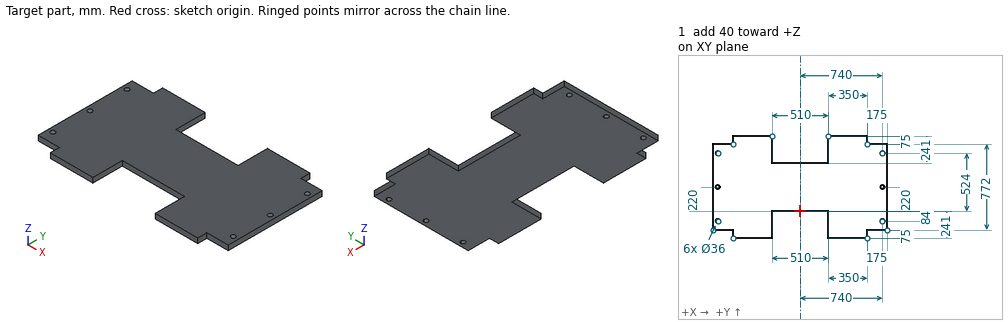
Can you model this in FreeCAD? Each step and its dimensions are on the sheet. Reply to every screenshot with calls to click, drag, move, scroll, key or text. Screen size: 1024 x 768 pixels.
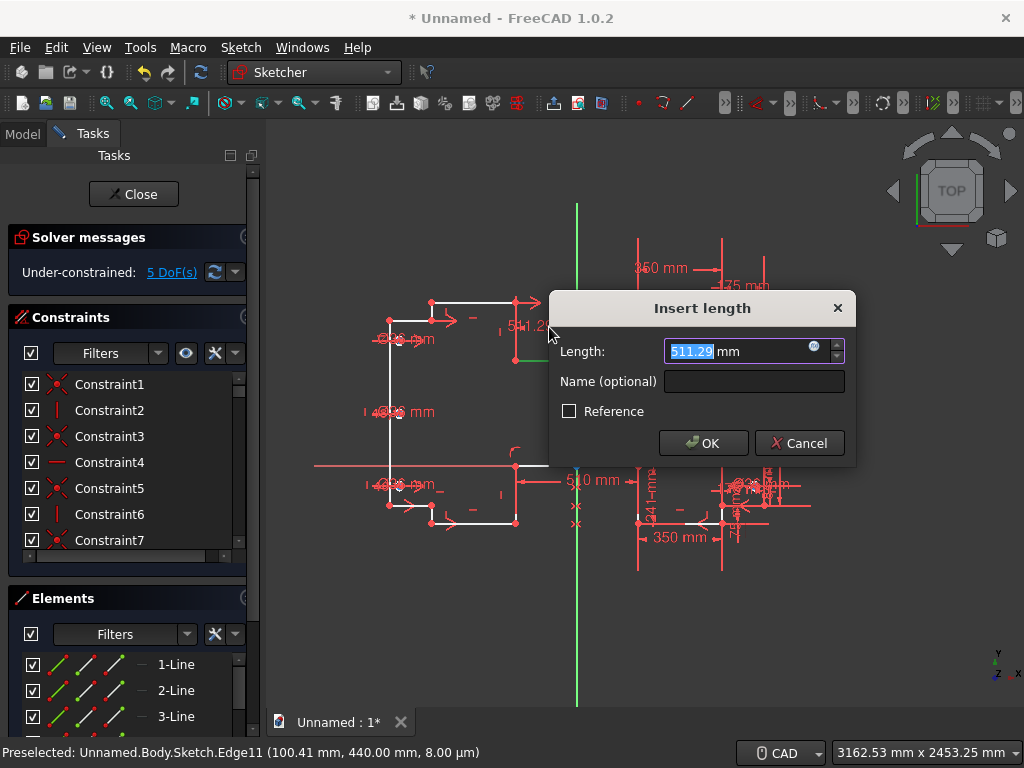
text(510)
key(Return)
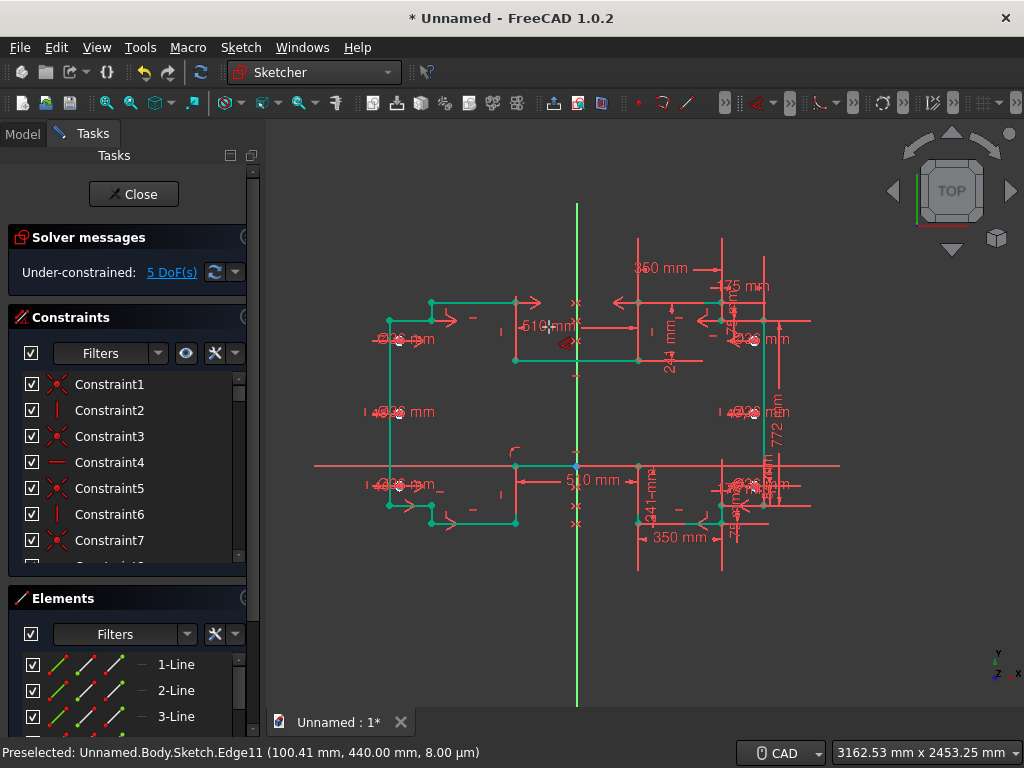
click(754, 486)
click(604, 520)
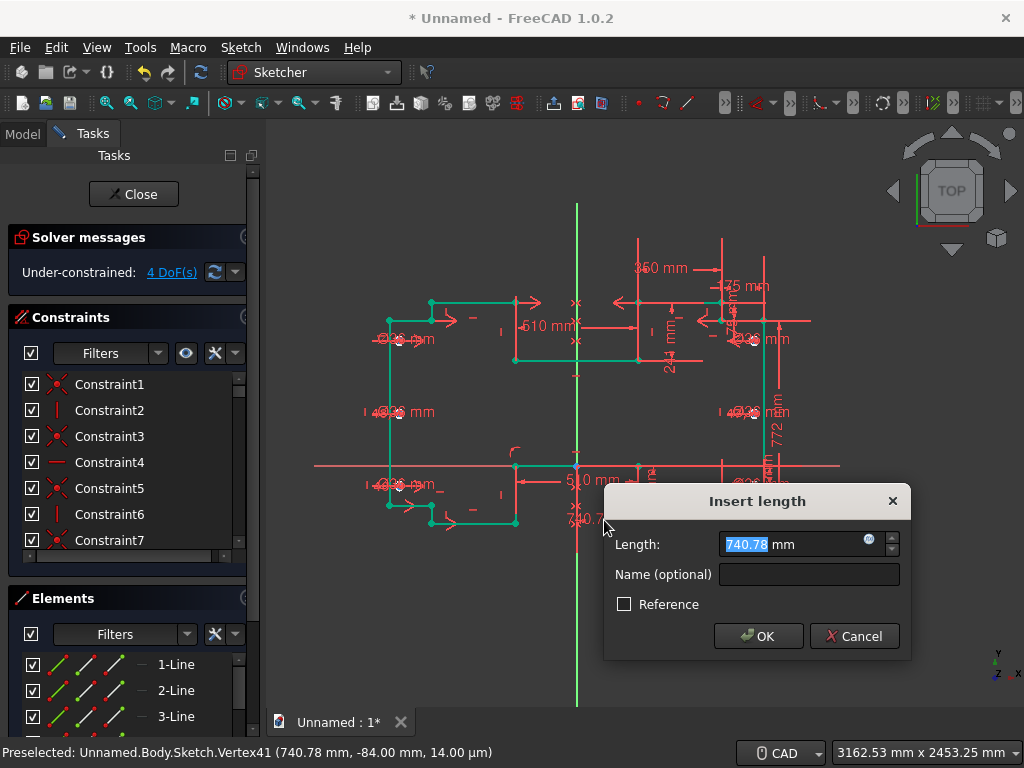
text(740)
key(Return)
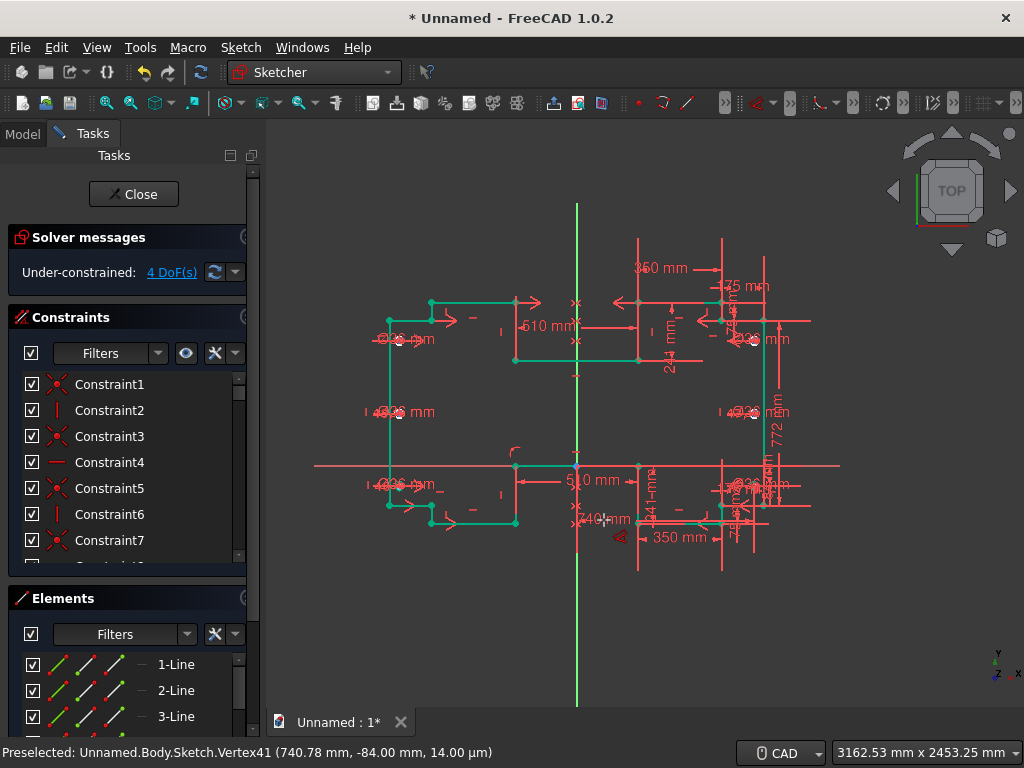
click(754, 414)
click(788, 452)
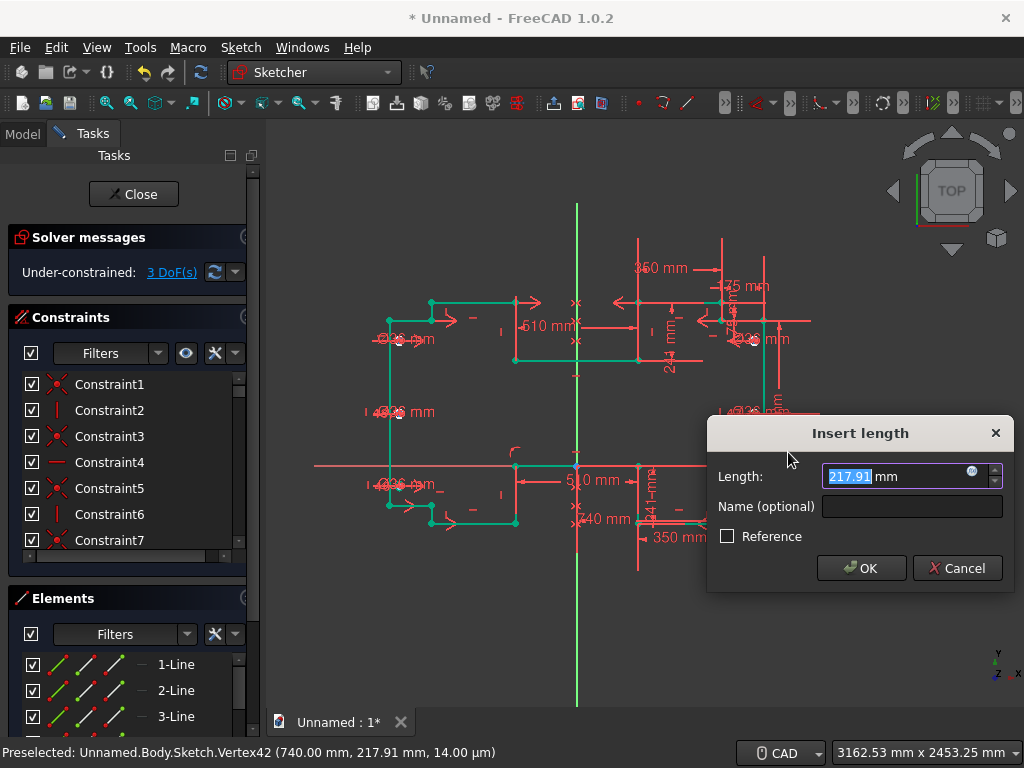
text(220)
key(Return)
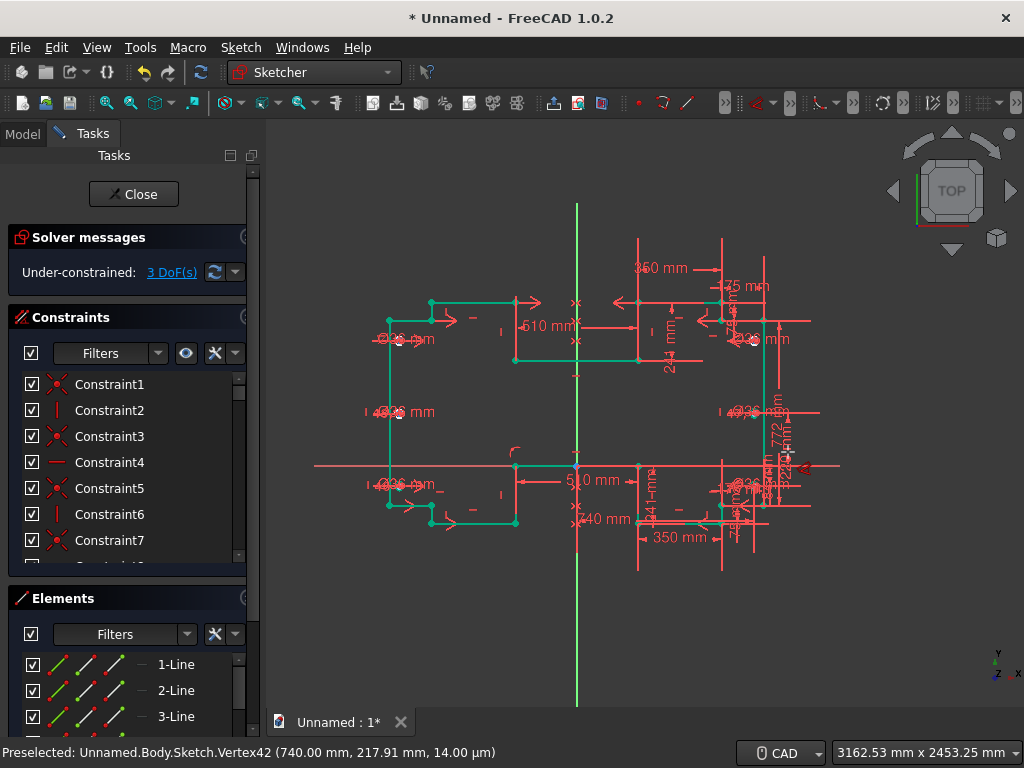
click(400, 414)
click(366, 440)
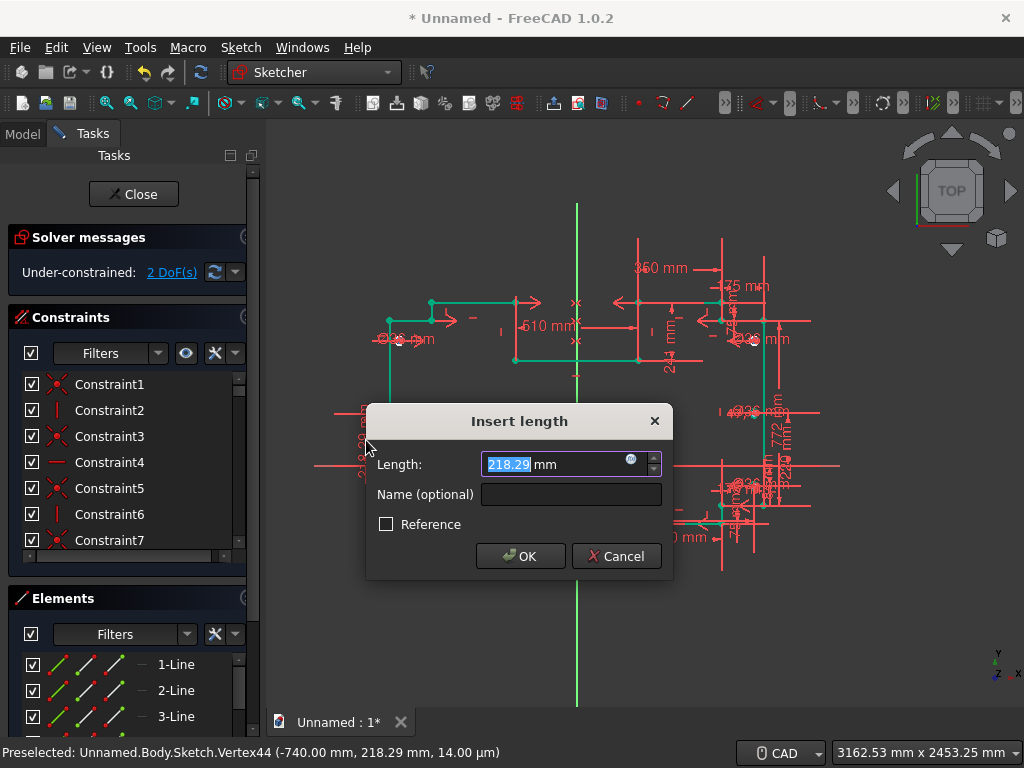
text(220)
key(Return)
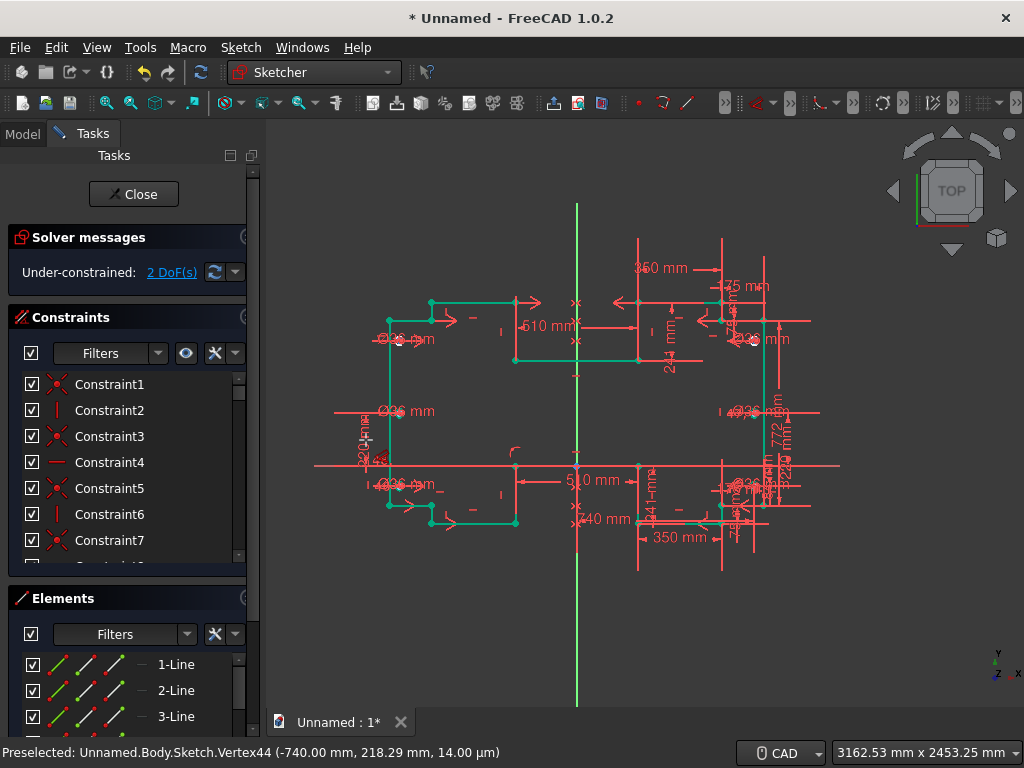
click(754, 341)
click(625, 307)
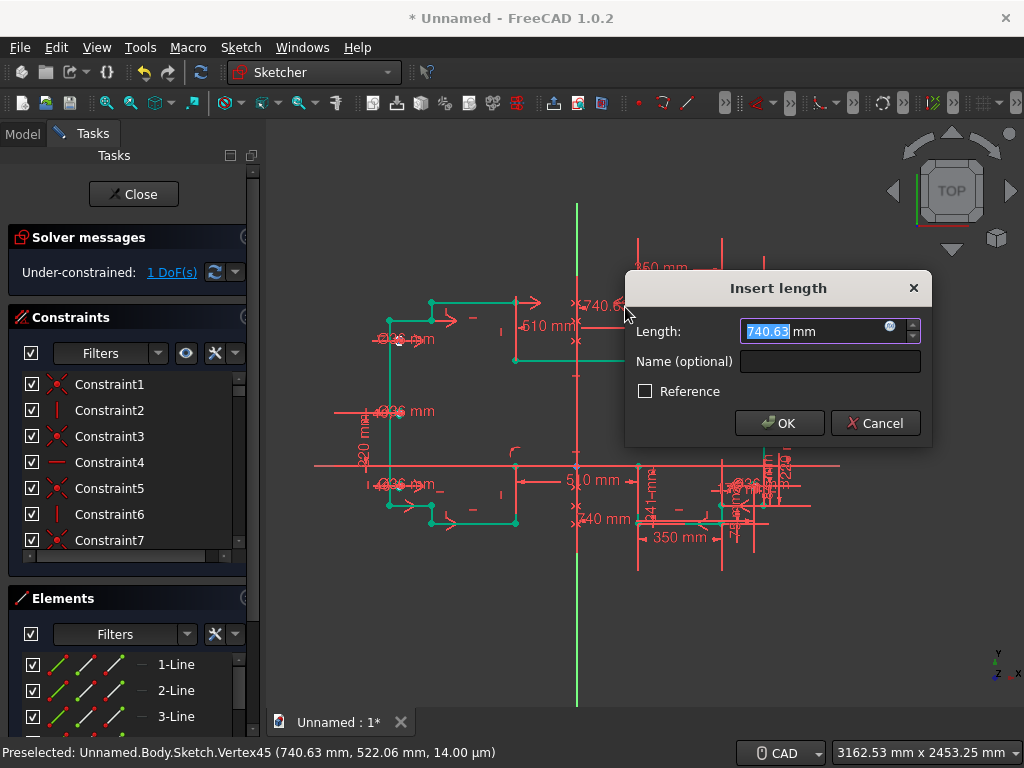
text(740)
key(Return)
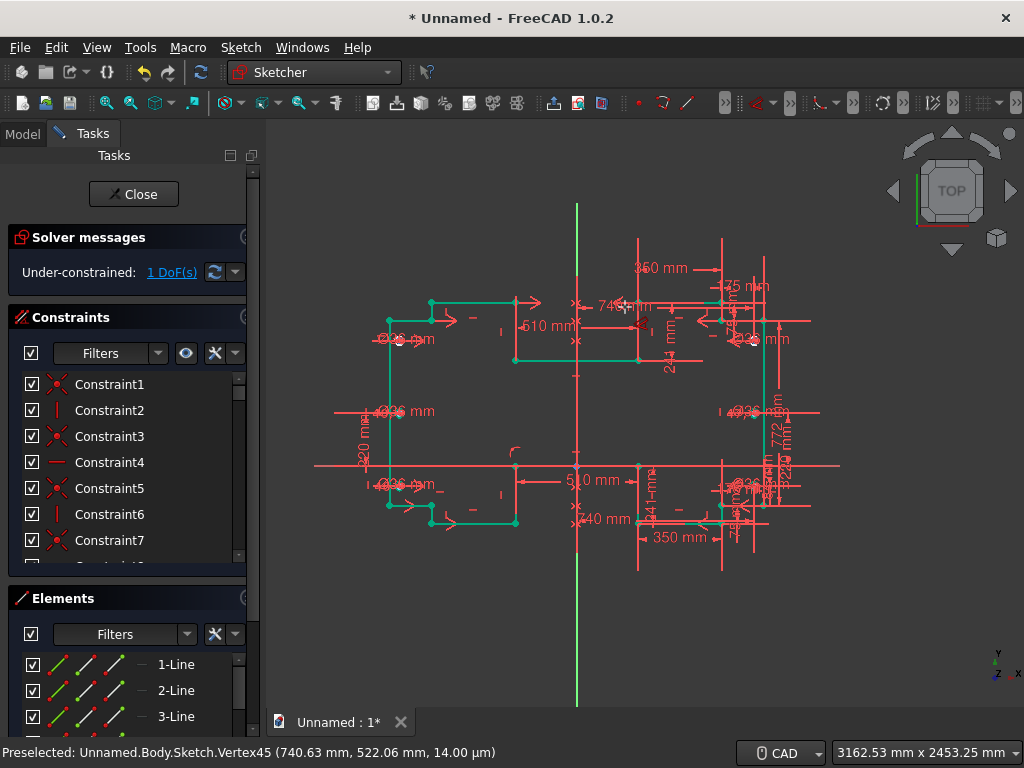
click(754, 341)
click(788, 375)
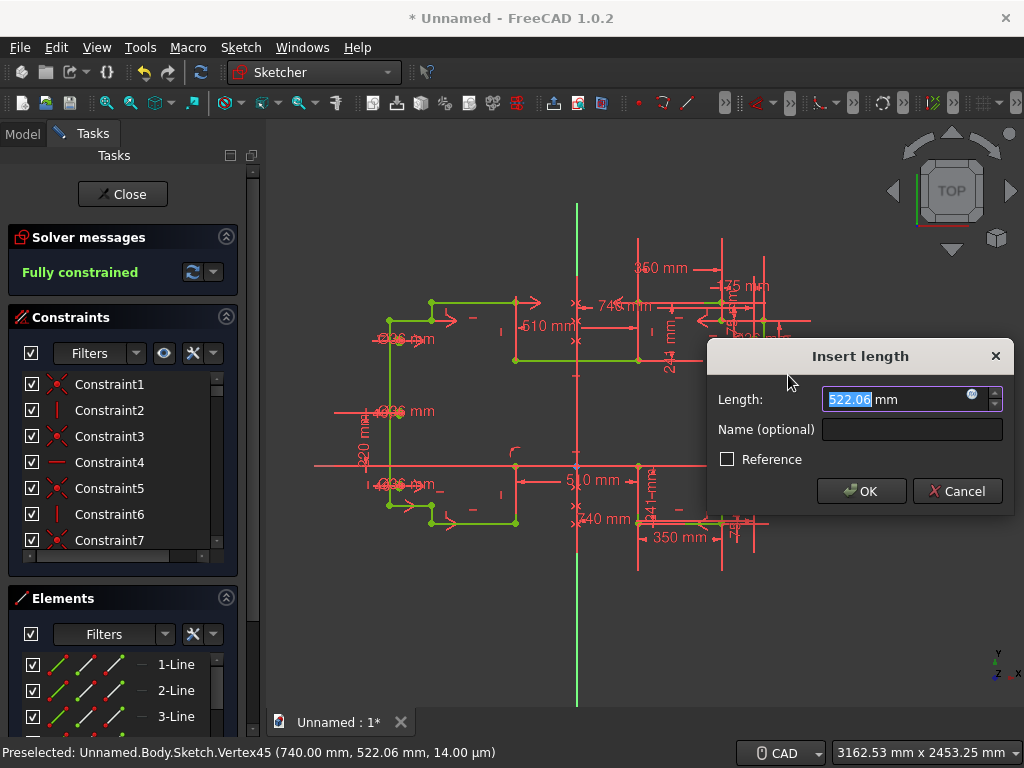
text(524)
key(Return)
key(Escape)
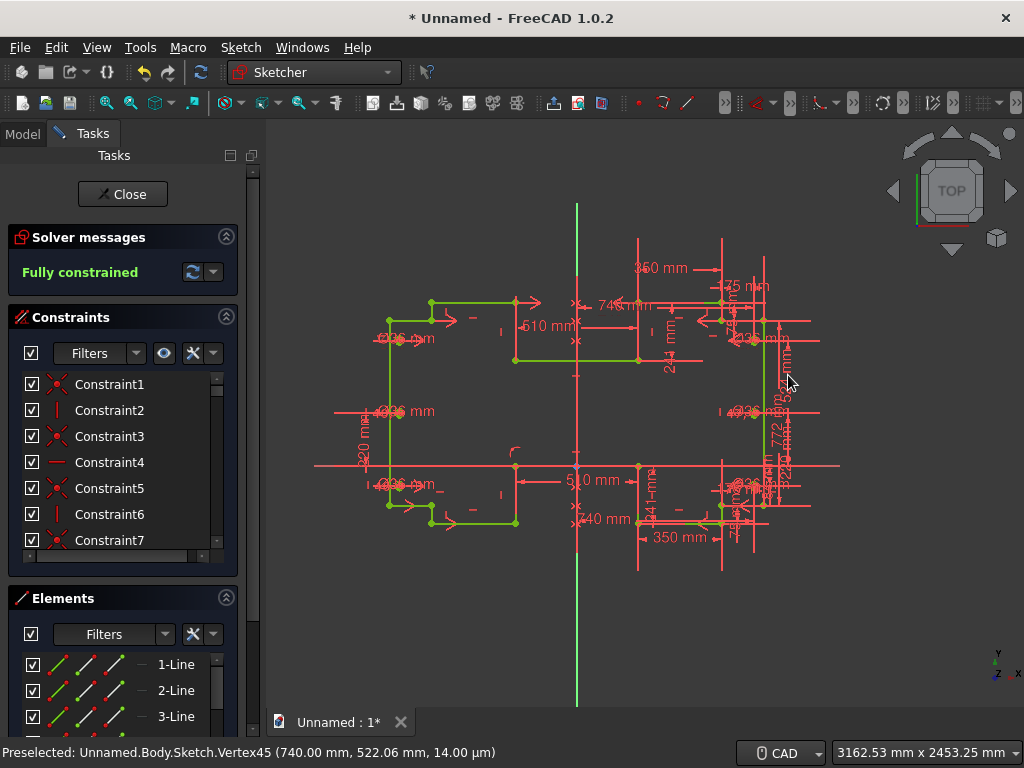
click(123, 194)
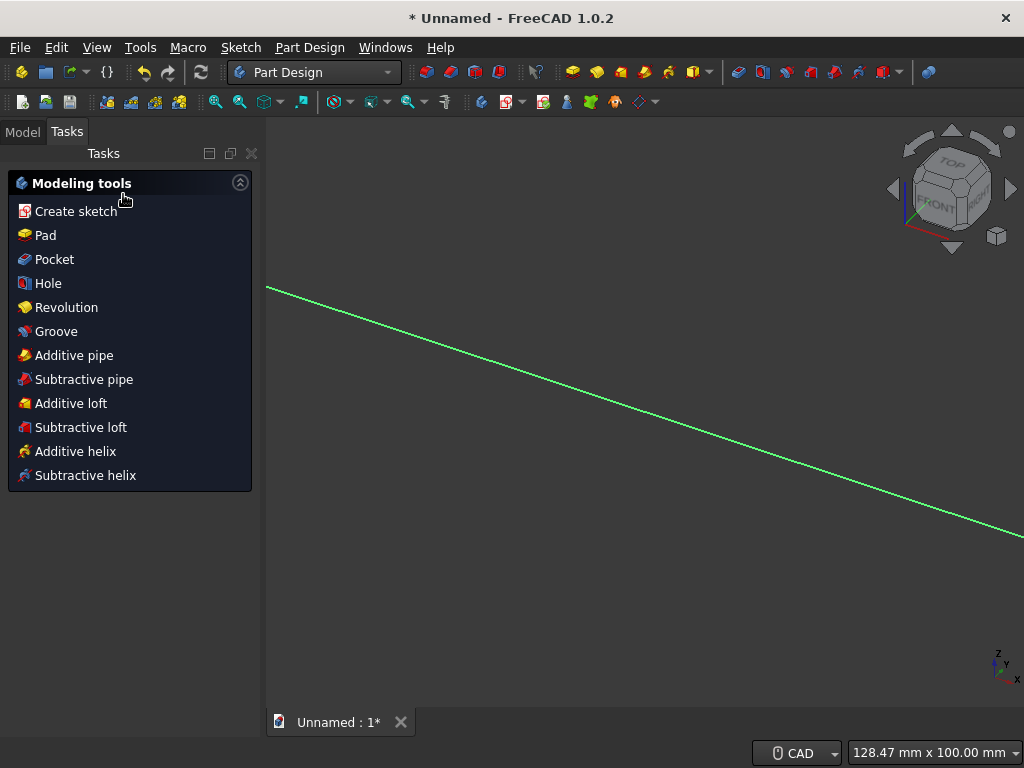
click(574, 72)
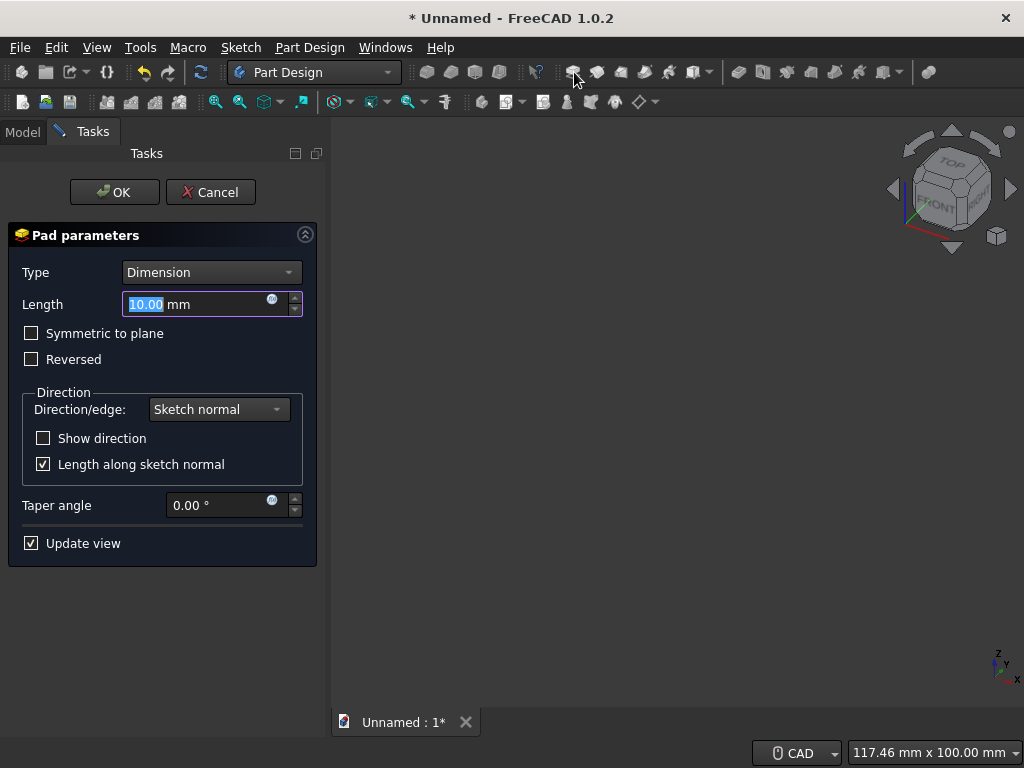
text(40)
key(Tab)